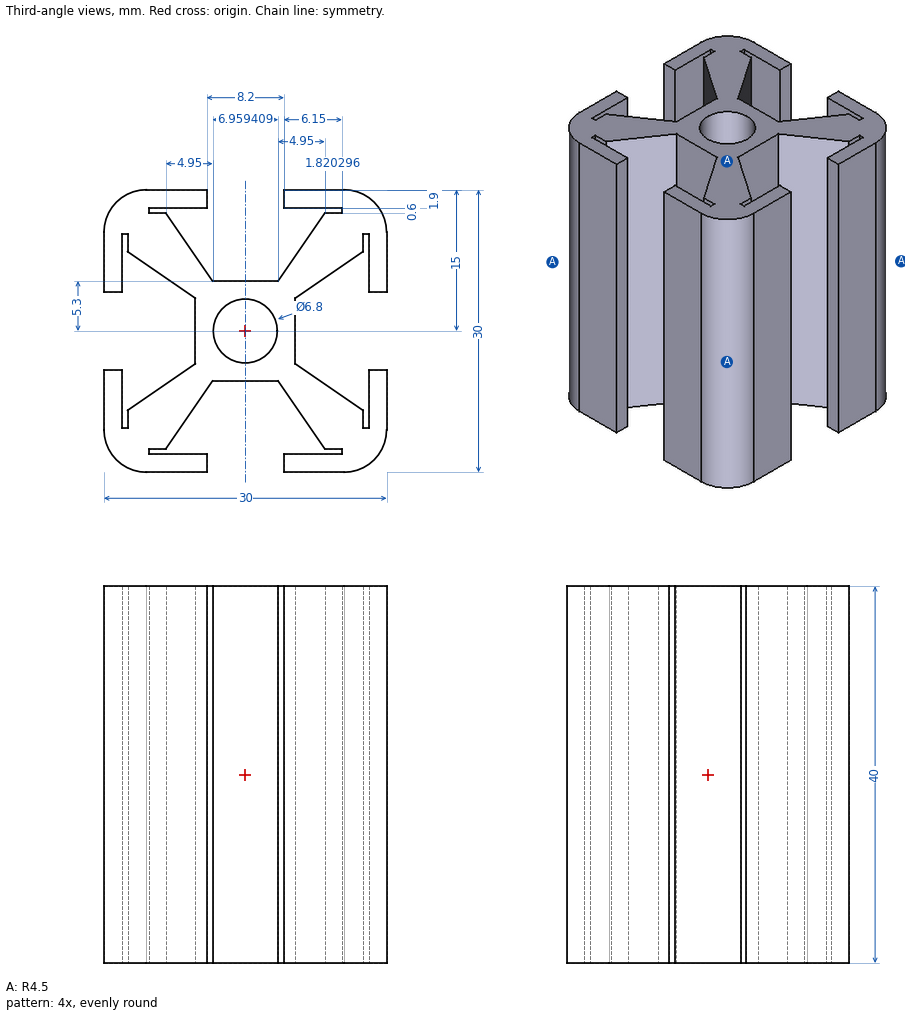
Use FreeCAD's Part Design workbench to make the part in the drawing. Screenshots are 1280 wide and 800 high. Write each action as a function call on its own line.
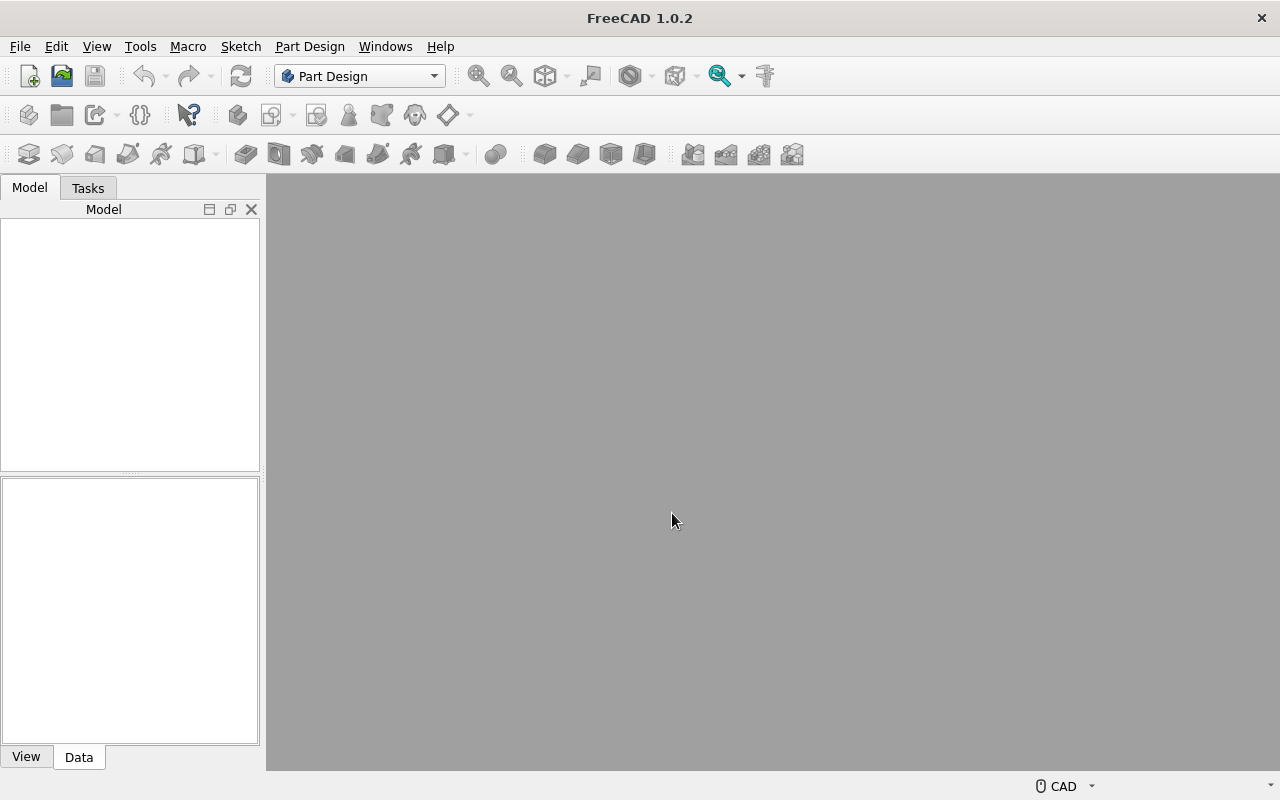
key(ctrl+n)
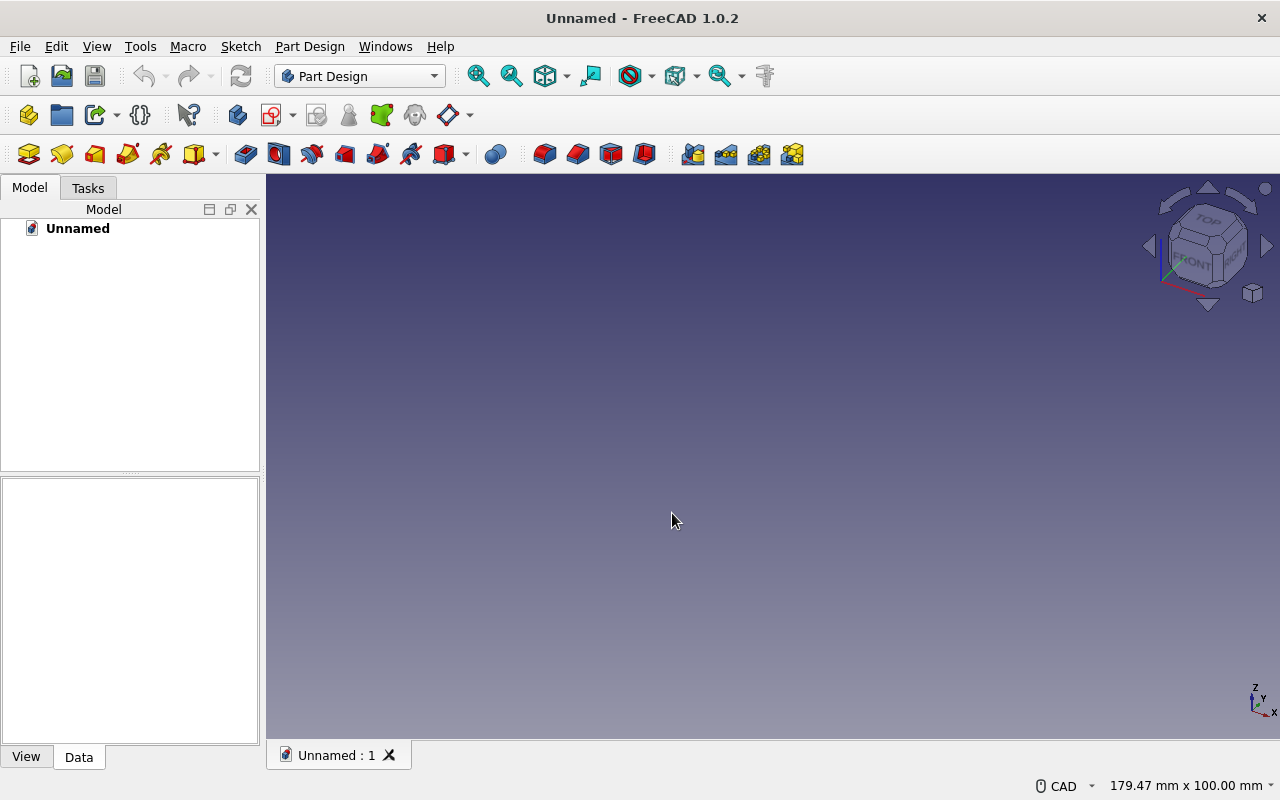
click(270, 116)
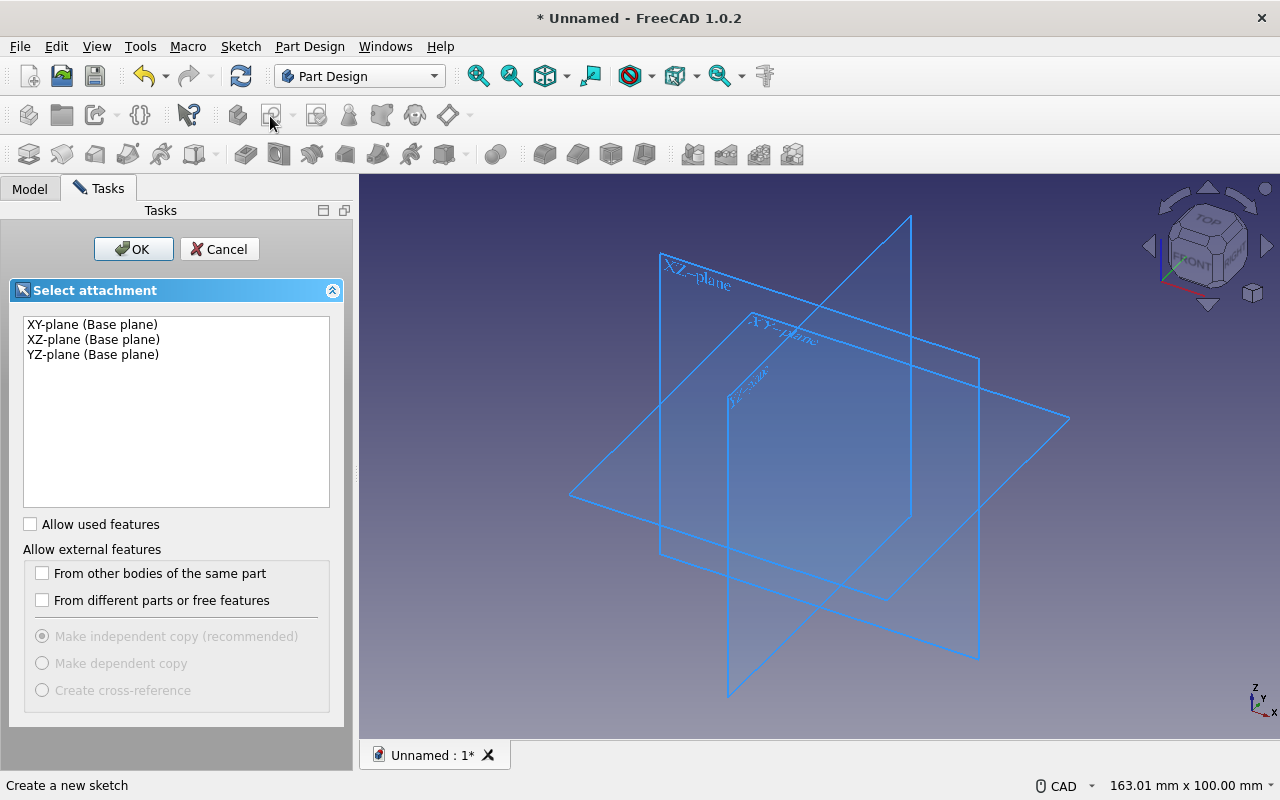
click(84, 324)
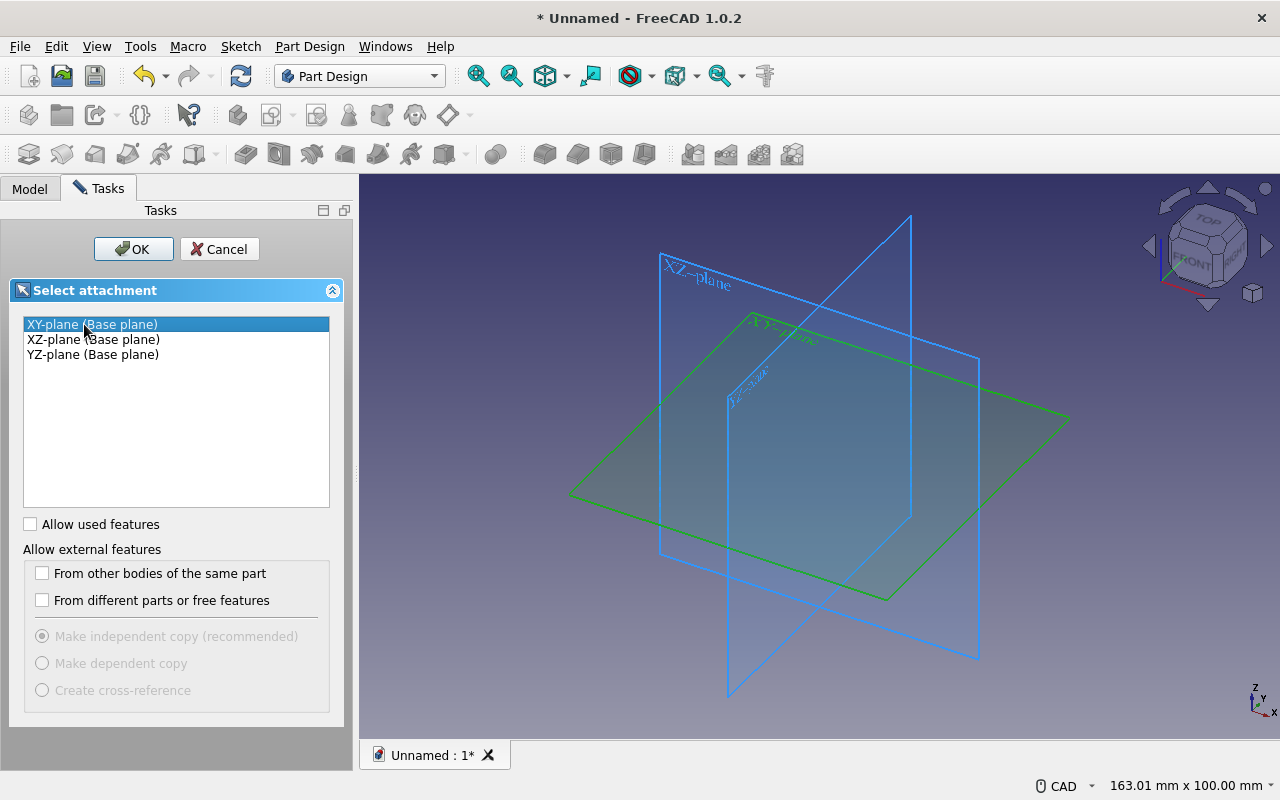
click(134, 249)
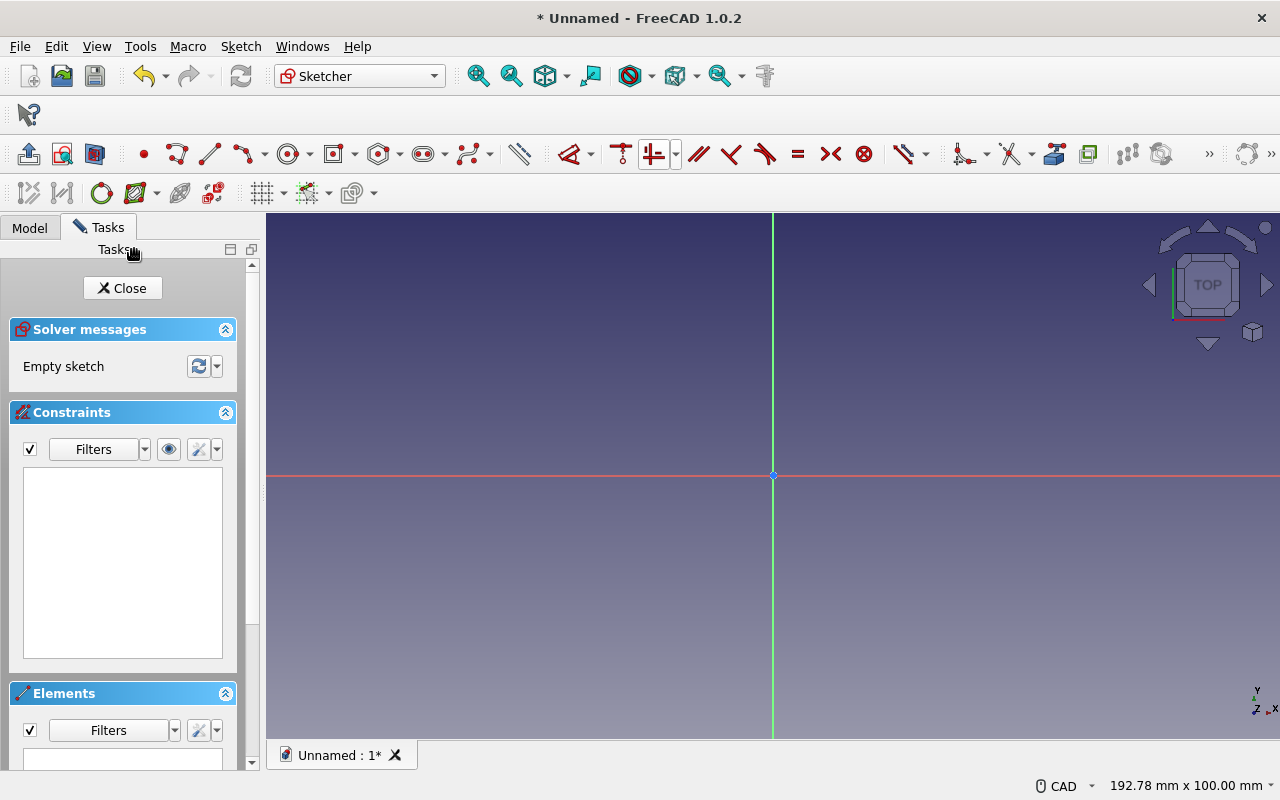
scroll(829, 476, up, 4)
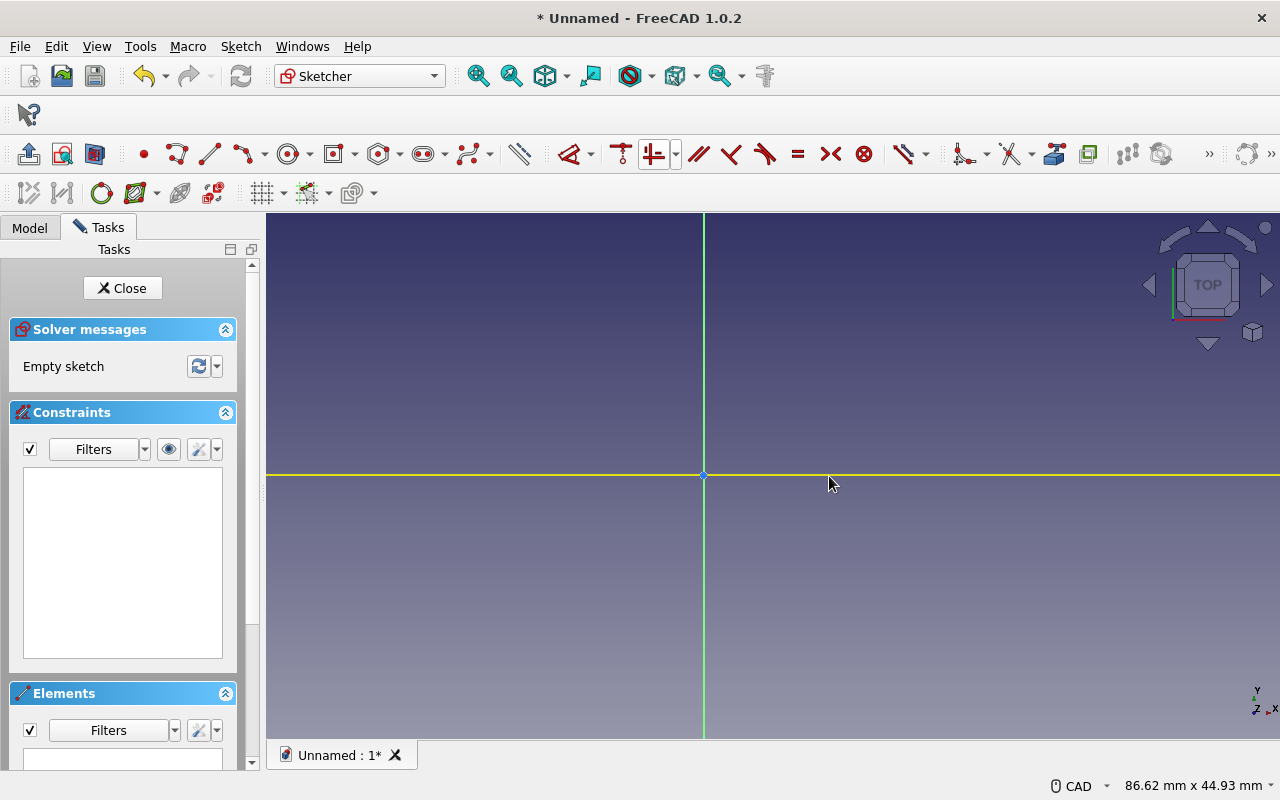
key(g)
key(v)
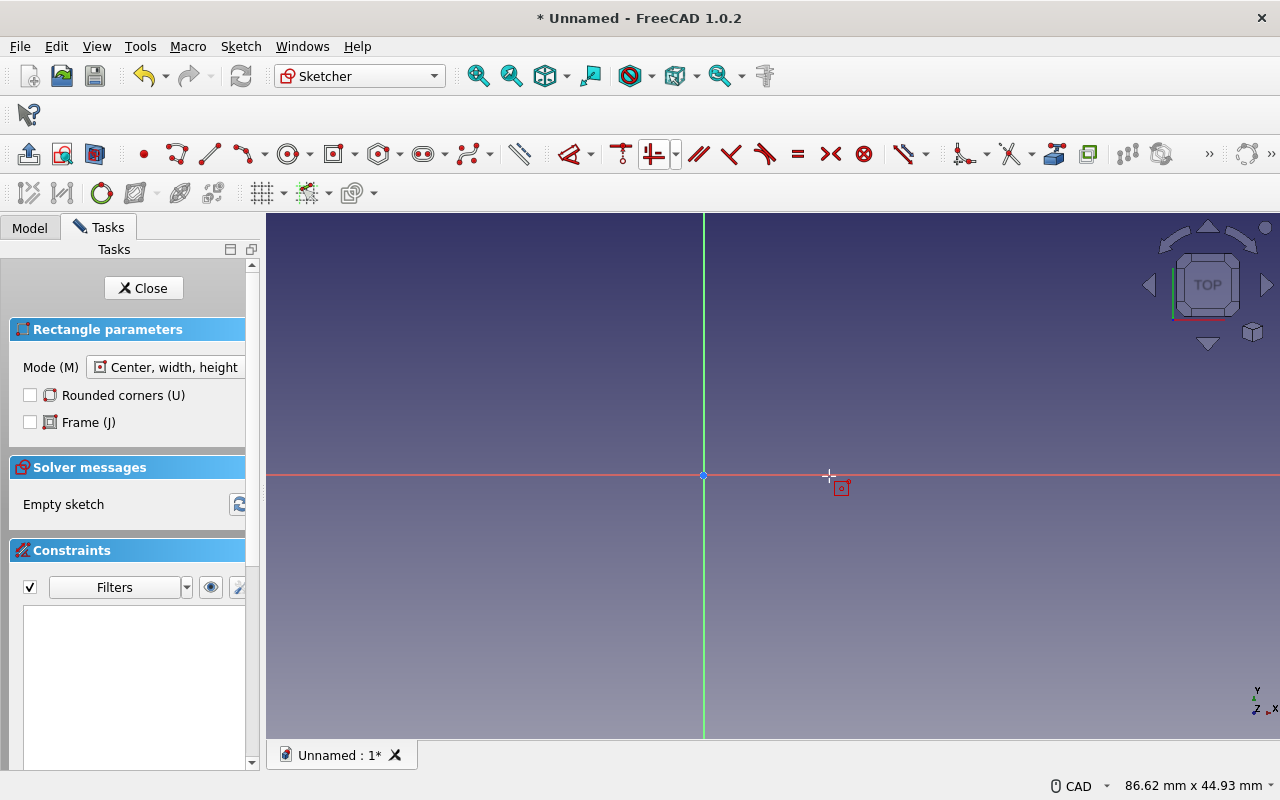
click(704, 475)
move(879, 300)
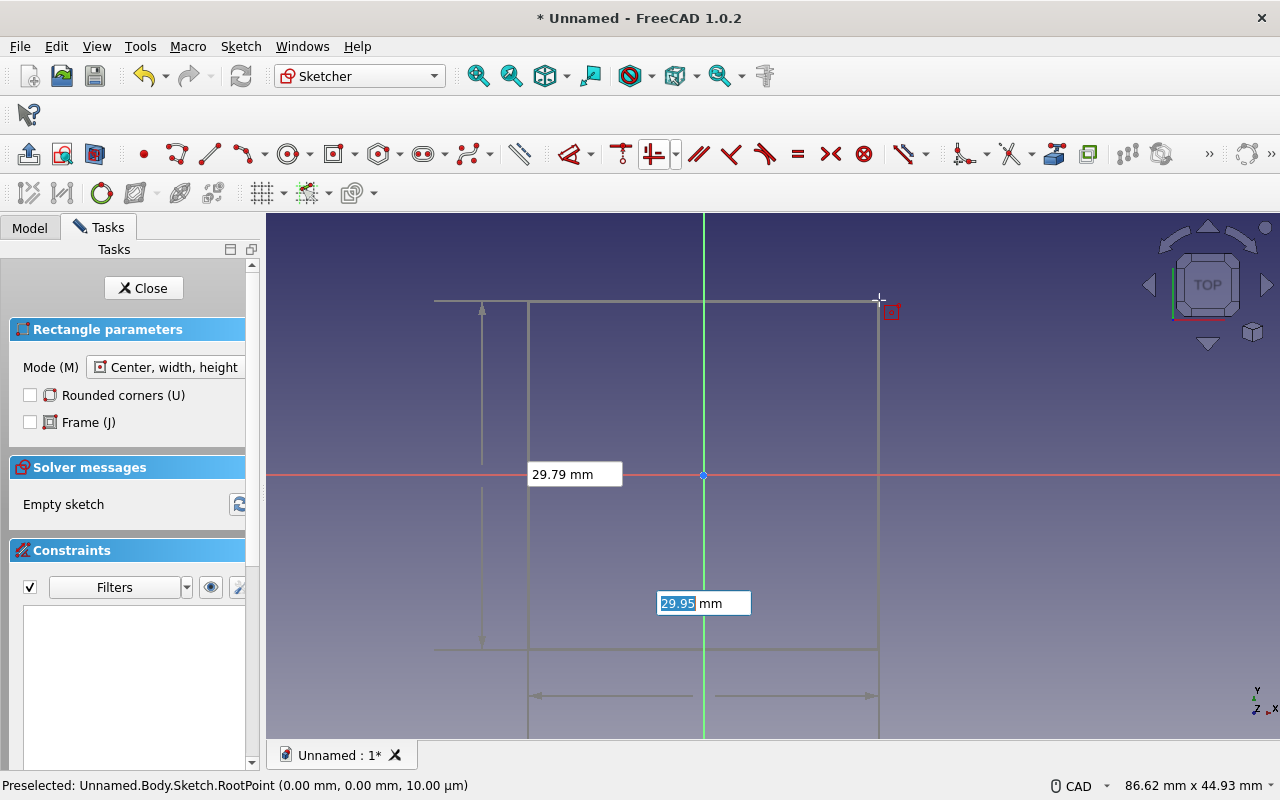
text(30)
key(Tab)
text(30)
key(Return)
key(Escape)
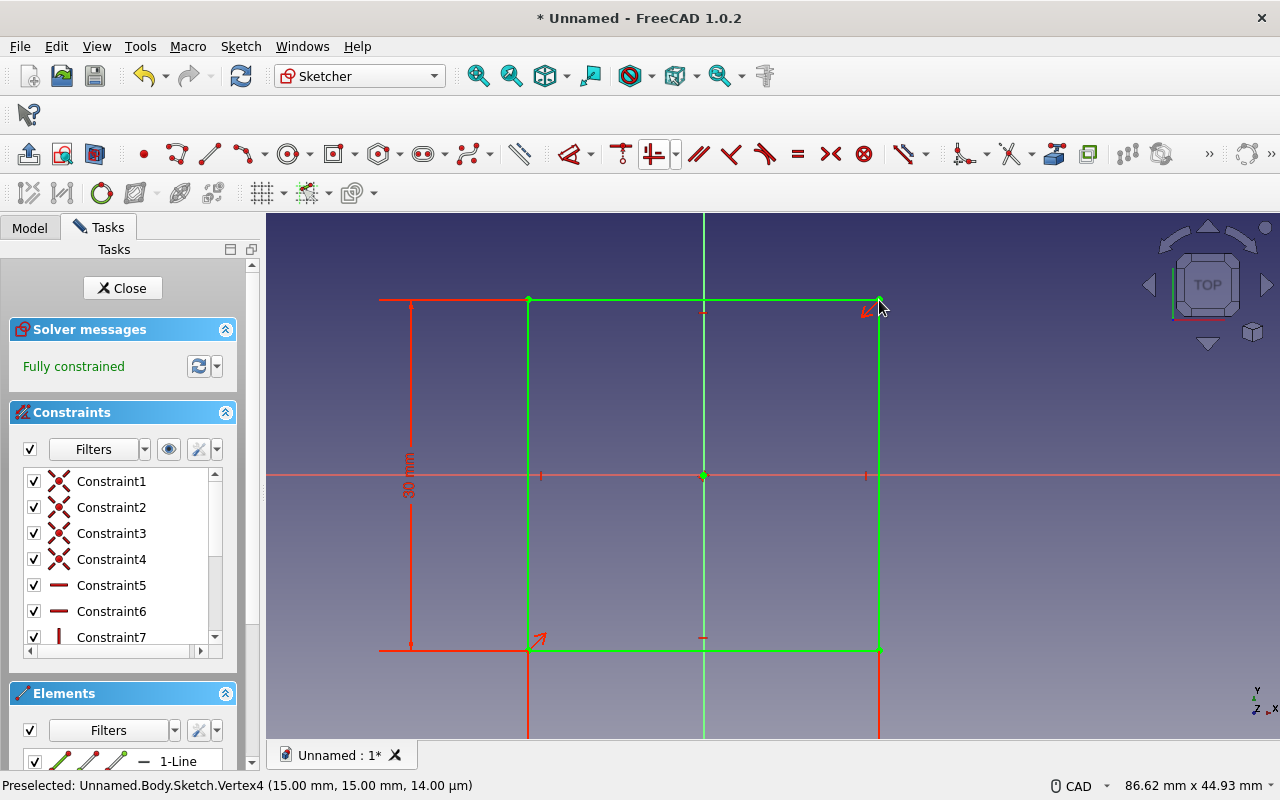
click(123, 288)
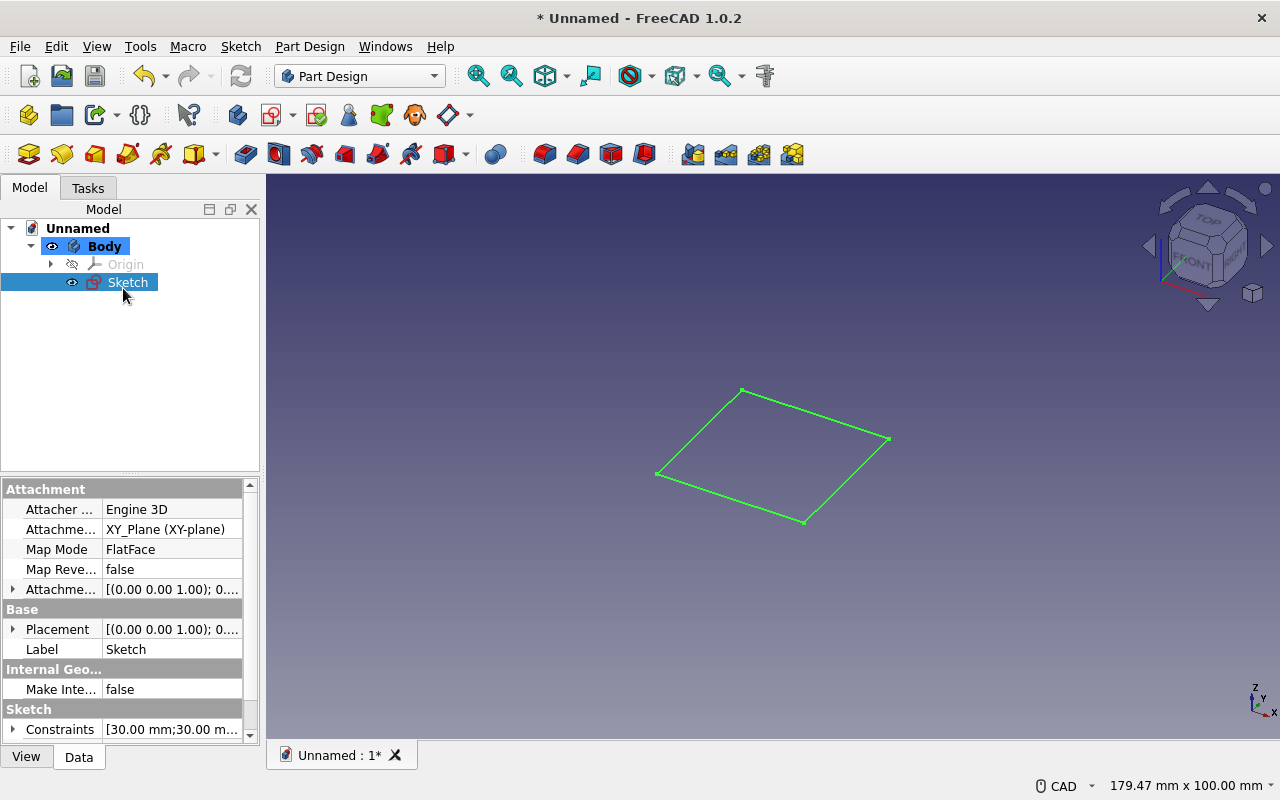
click(29, 154)